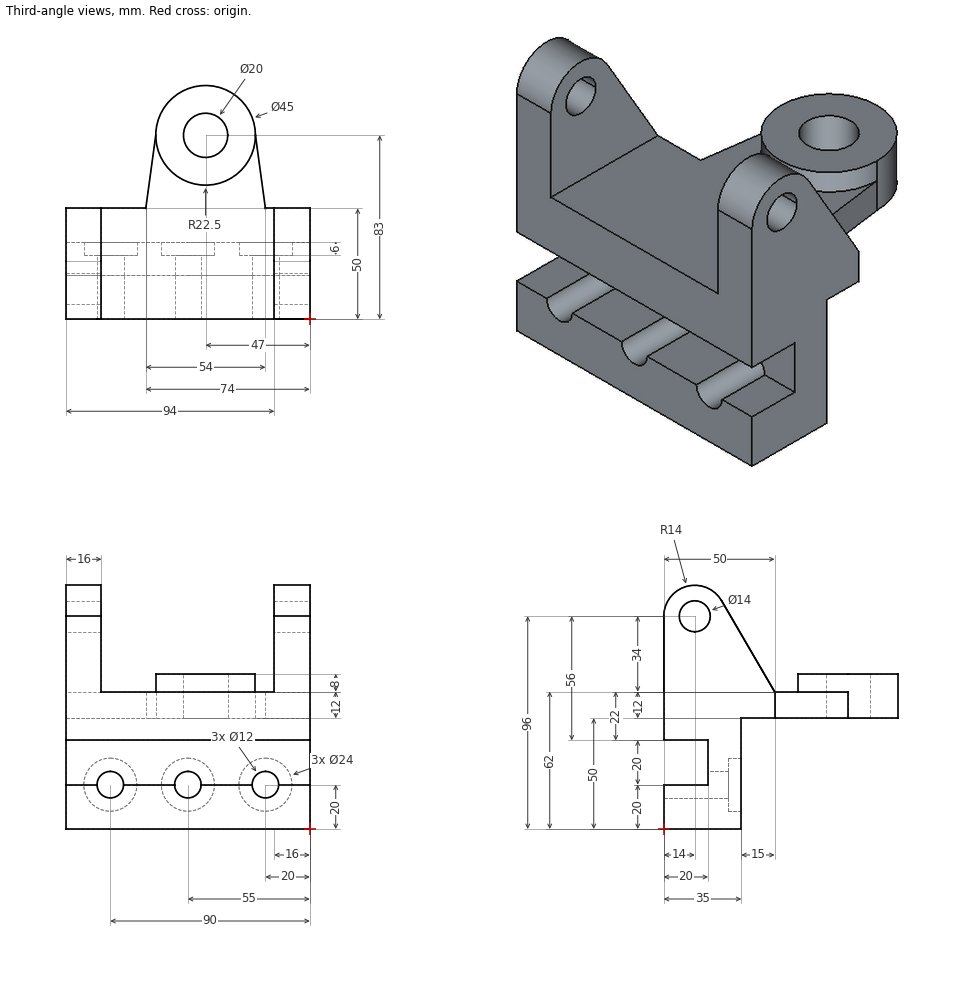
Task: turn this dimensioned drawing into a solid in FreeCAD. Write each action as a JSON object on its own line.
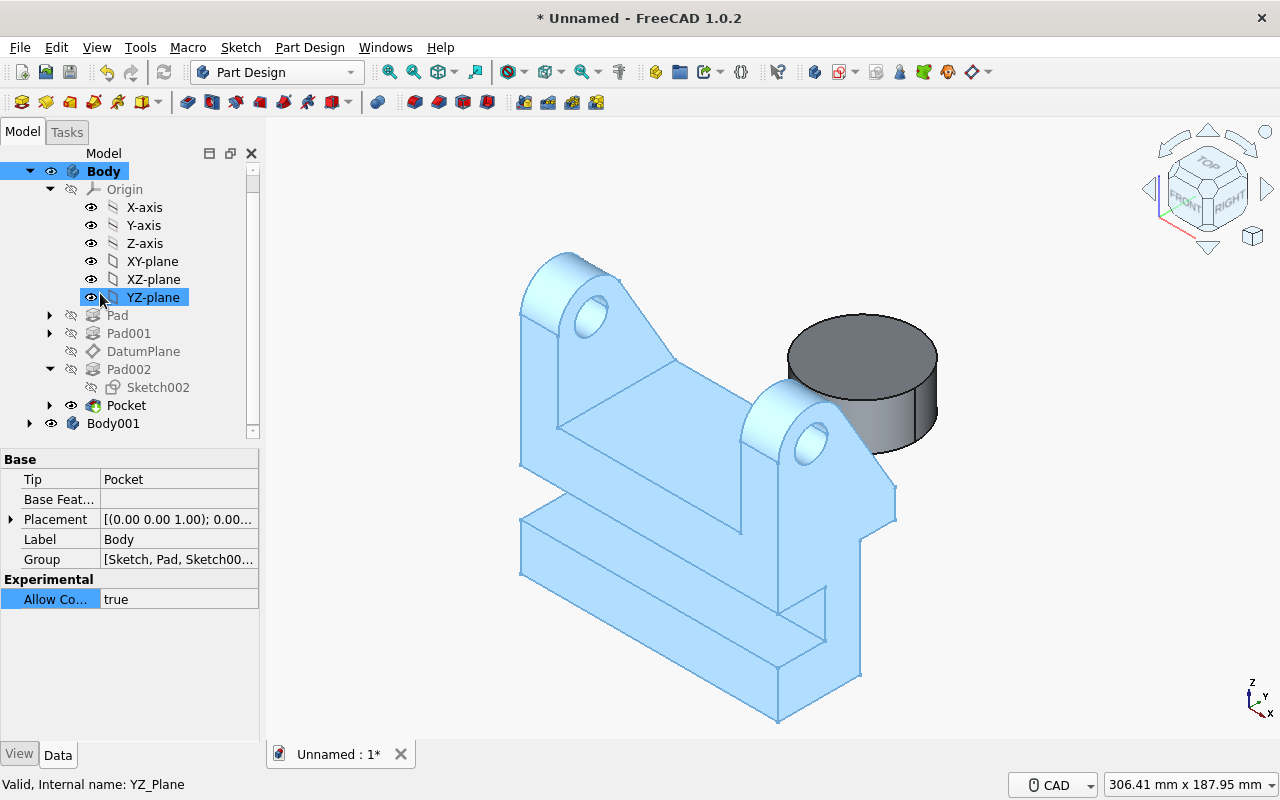
{"action": "left_click", "coordinate": [96, 423]}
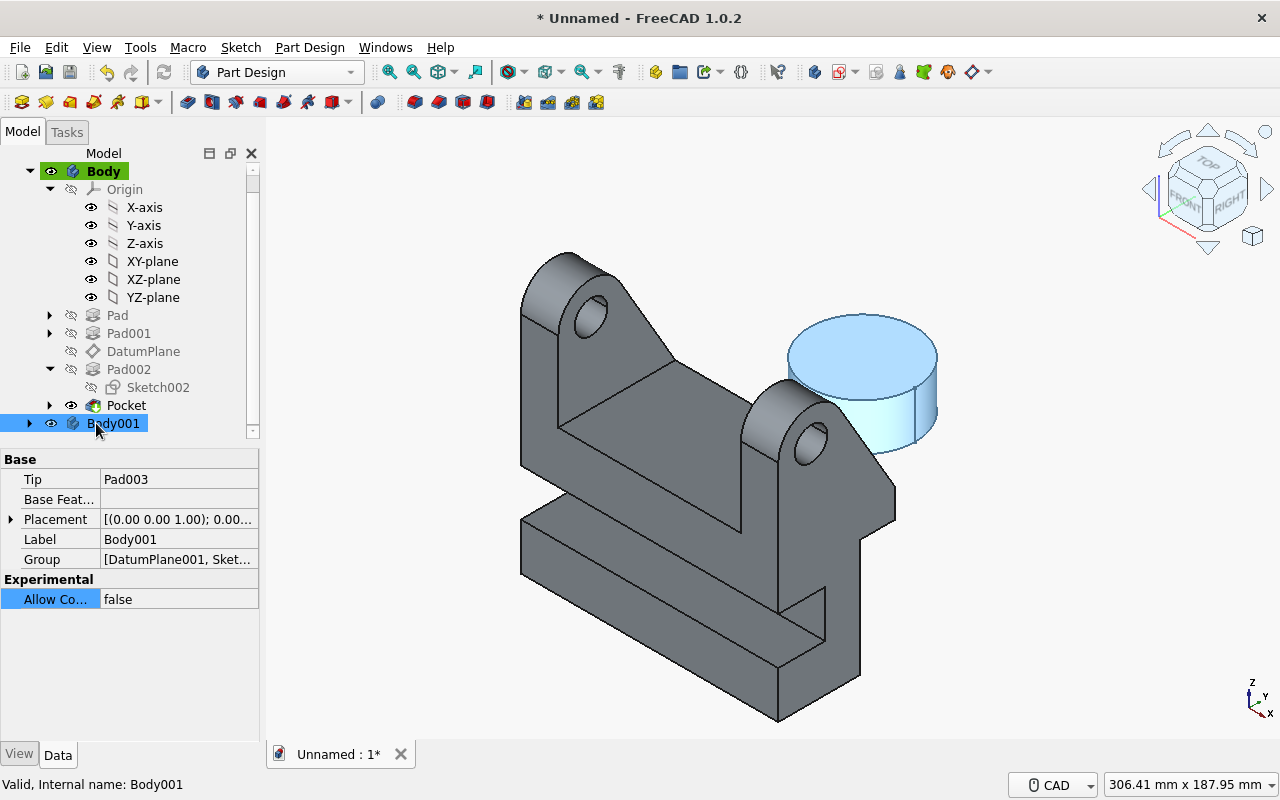
{"action": "left_click", "coordinate": [378, 102]}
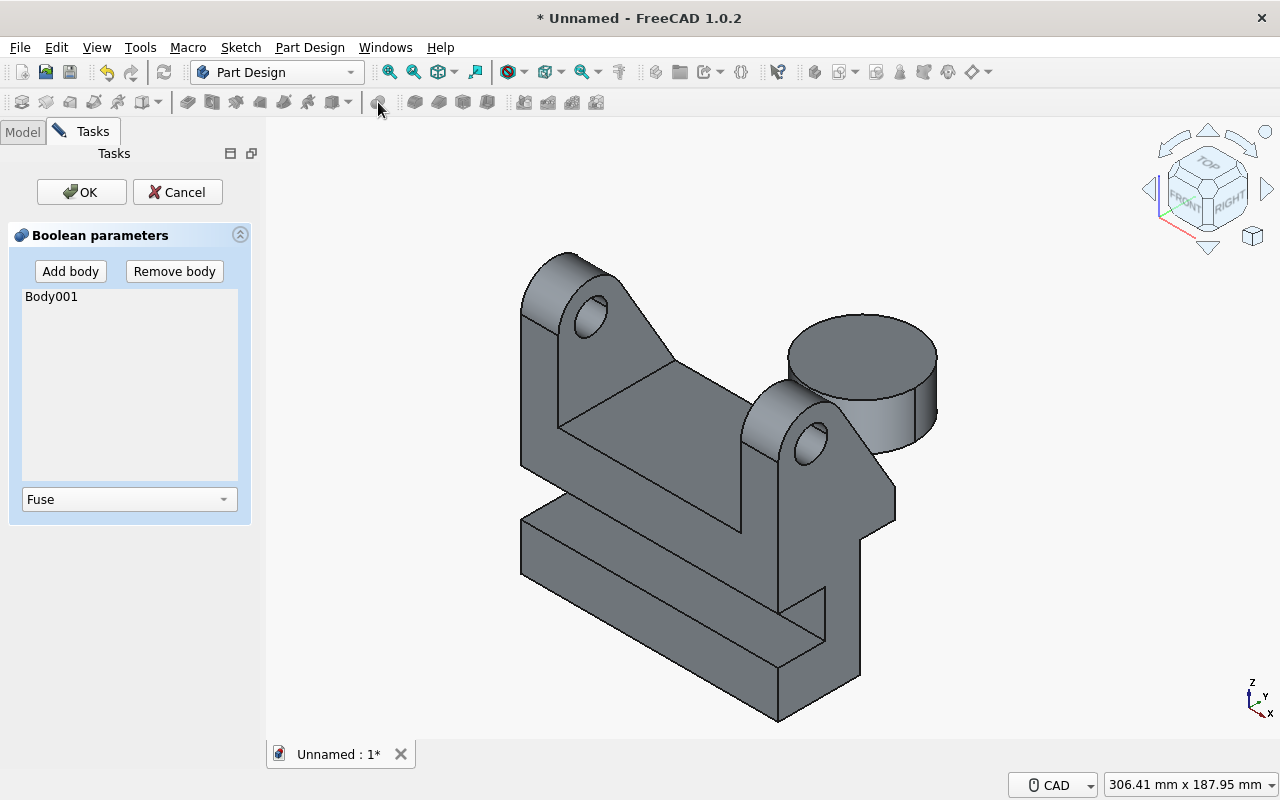
{"action": "left_click", "coordinate": [82, 192]}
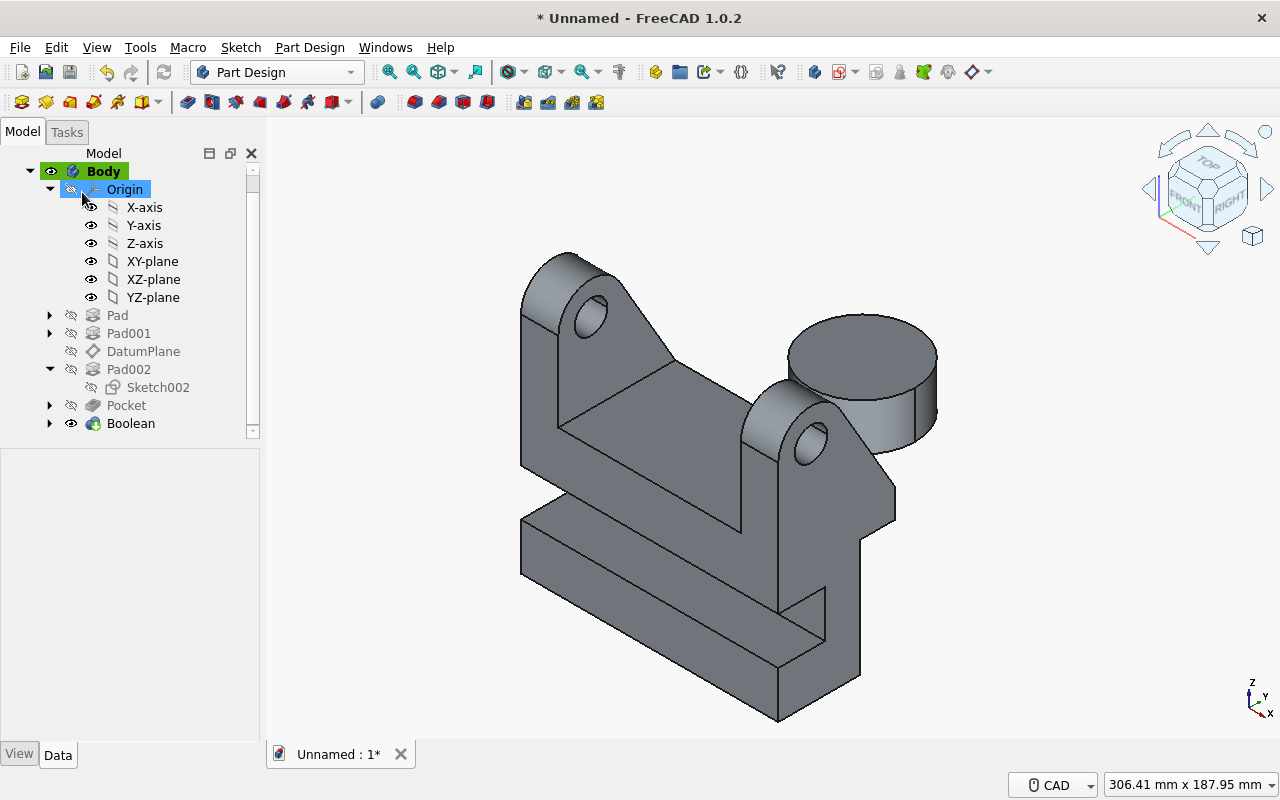
{"action": "left_click", "coordinate": [708, 446]}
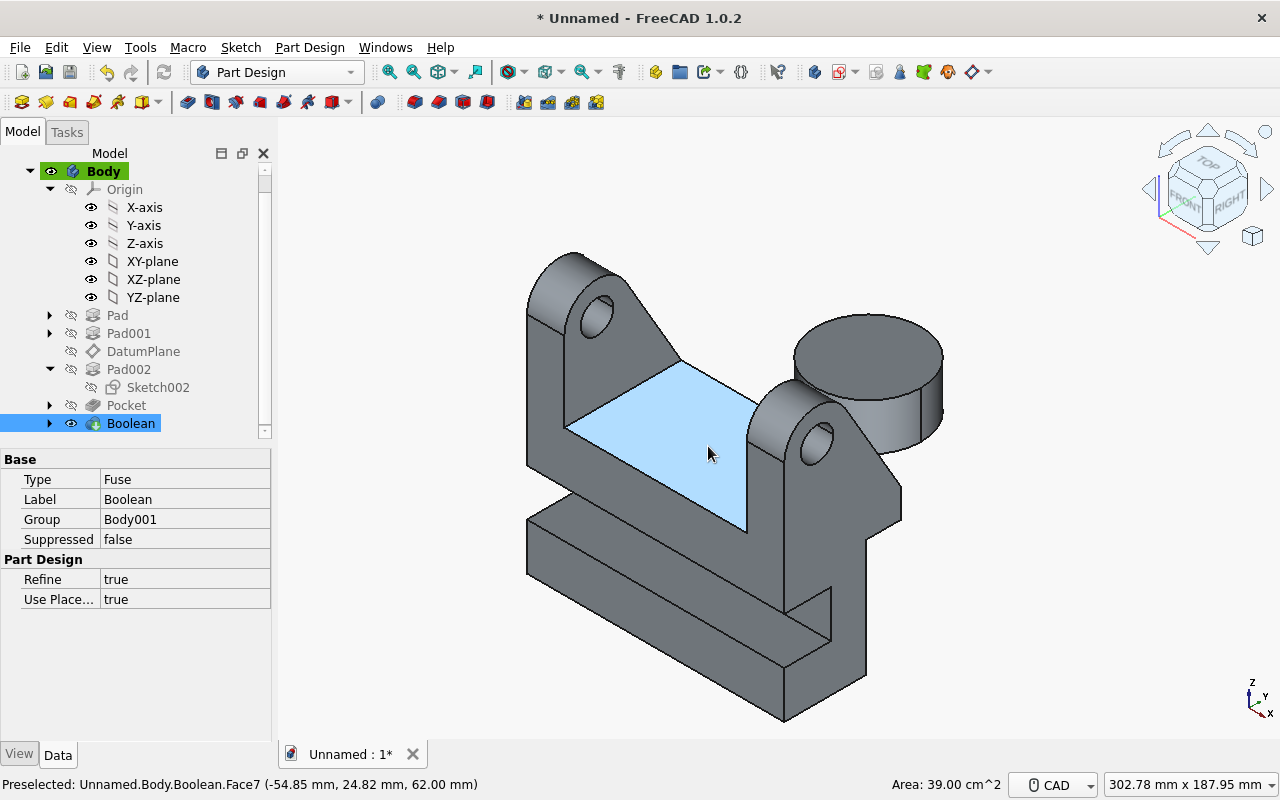
{"action": "left_click", "coordinate": [840, 72]}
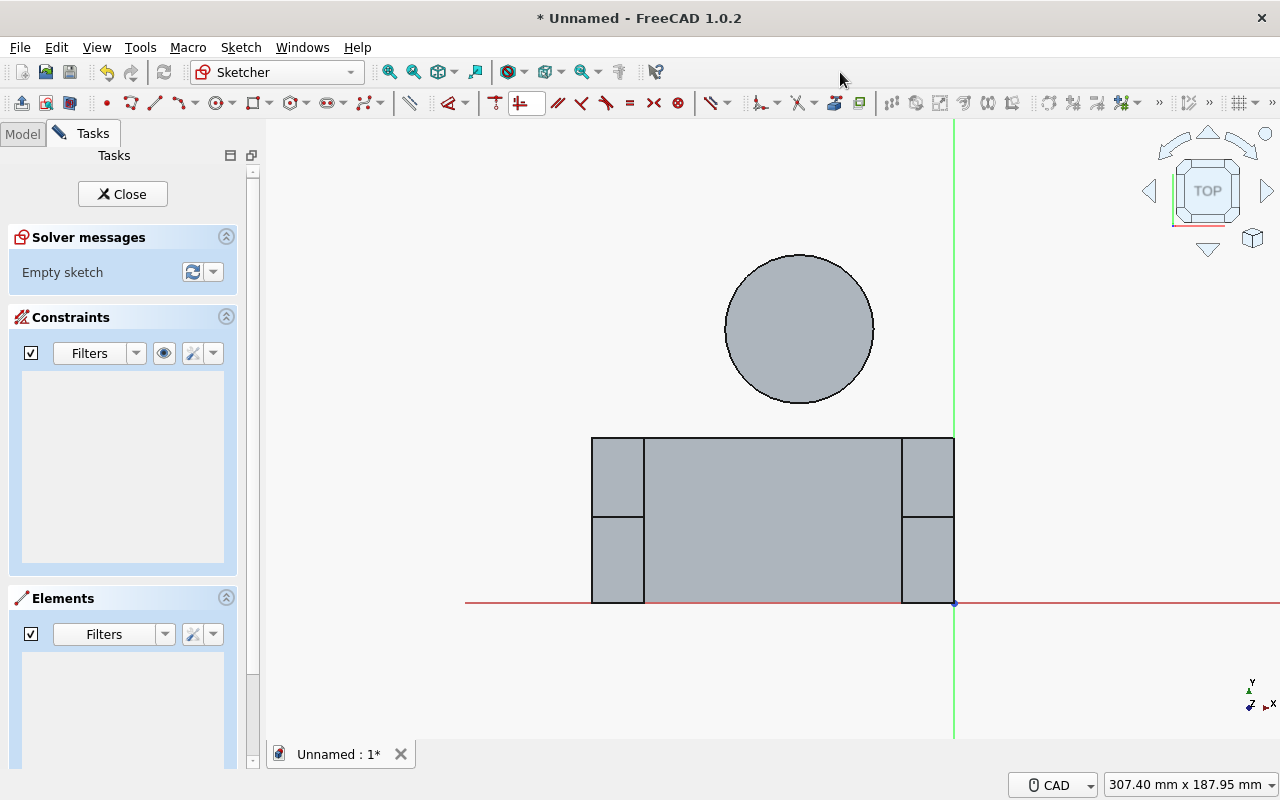
{"action": "left_click", "coordinate": [70, 104]}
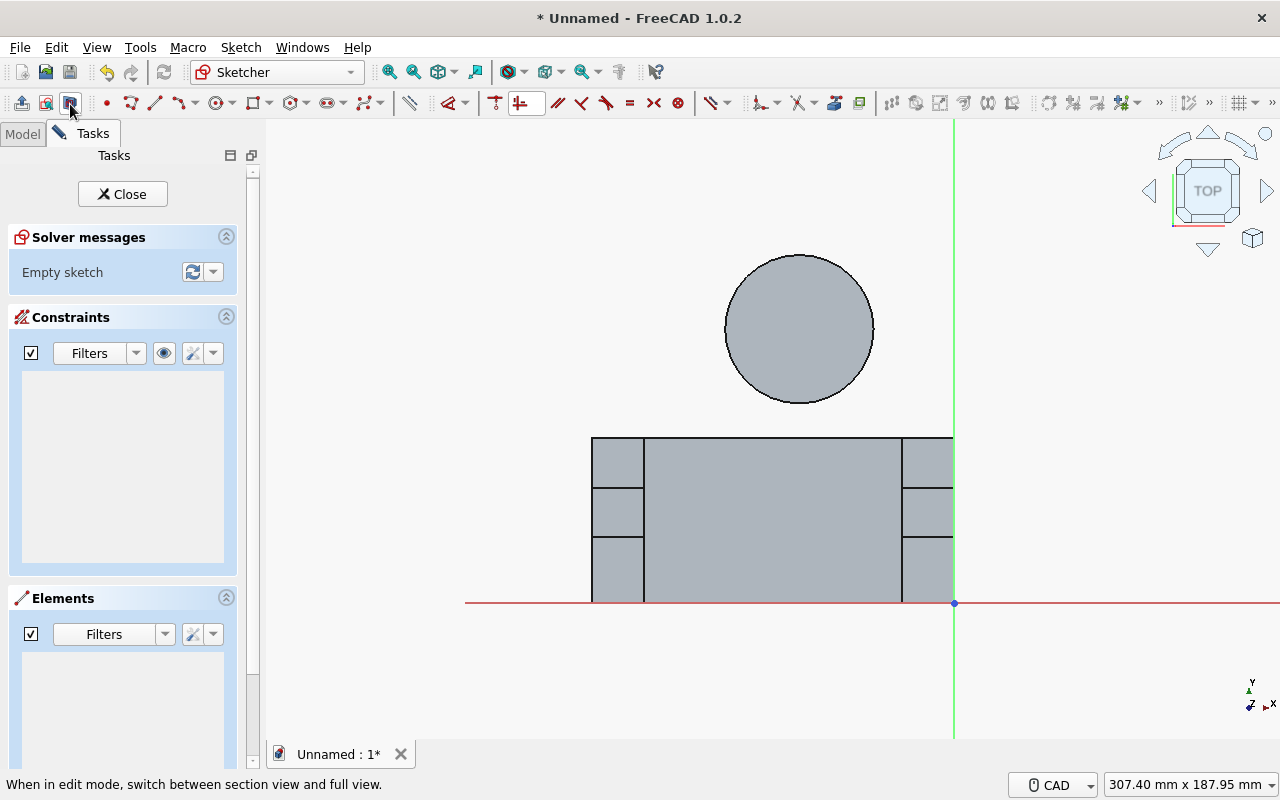
{"action": "scroll", "coordinate": [1092, 542], "scroll_direction": "up", "scroll_amount": 2}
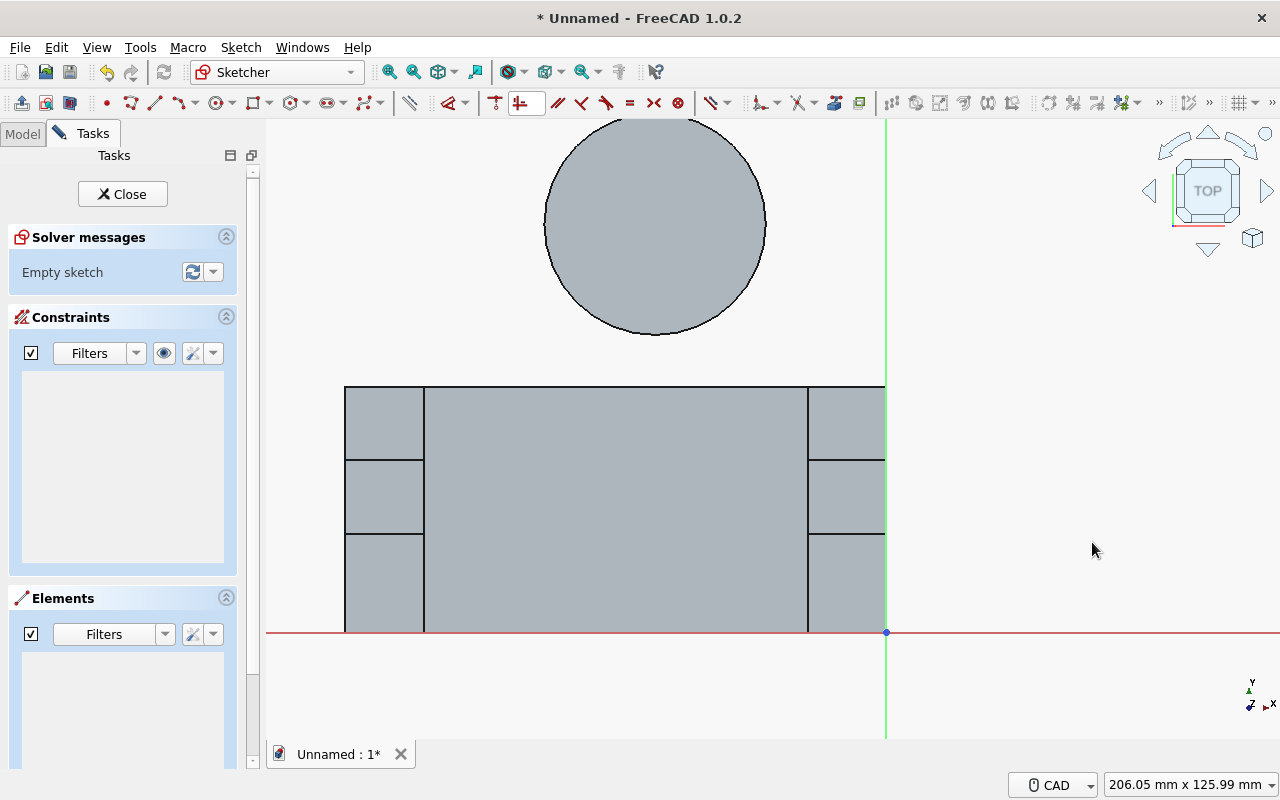
{"action": "left_click", "coordinate": [132, 104]}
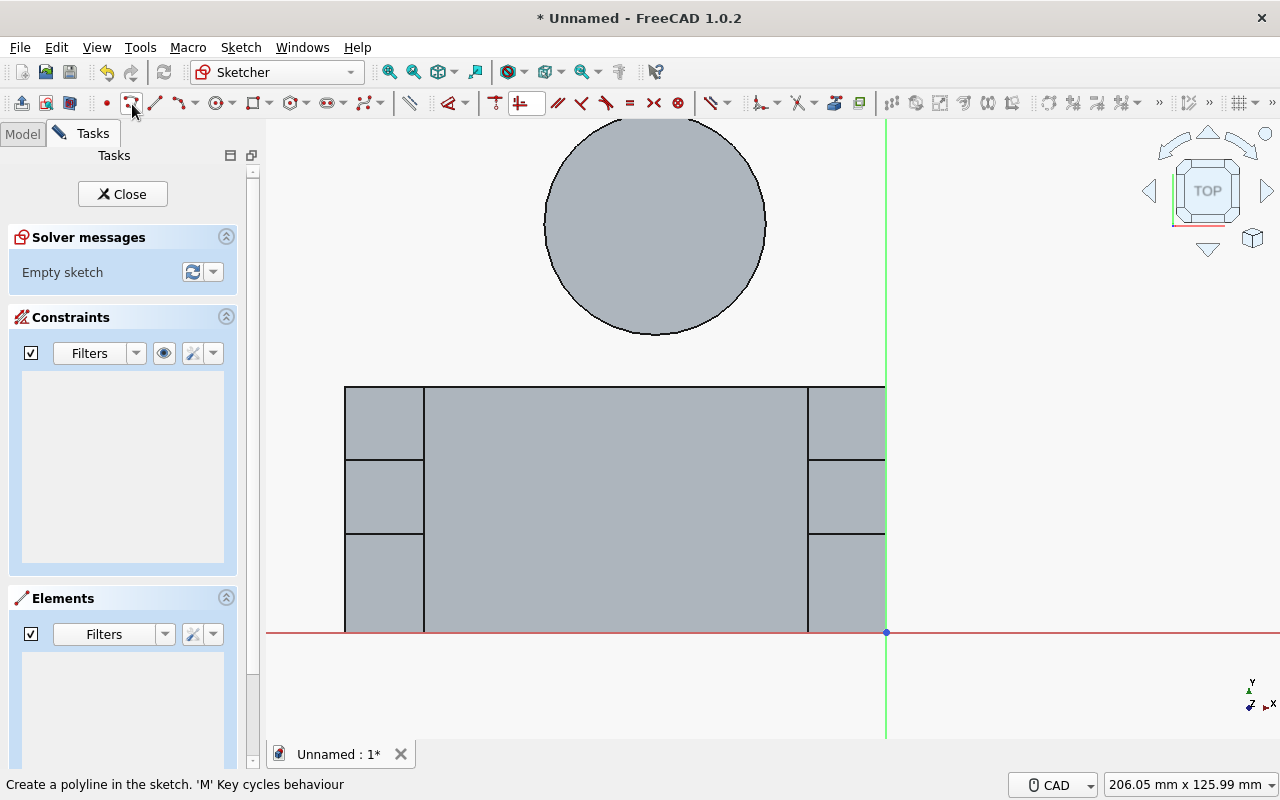
{"action": "left_click", "coordinate": [544, 224]}
{"action": "left_click", "coordinate": [522, 387]}
{"action": "left_click", "coordinate": [788, 387]}
{"action": "left_click", "coordinate": [766, 224]}
{"action": "right_click", "coordinate": [766, 224]}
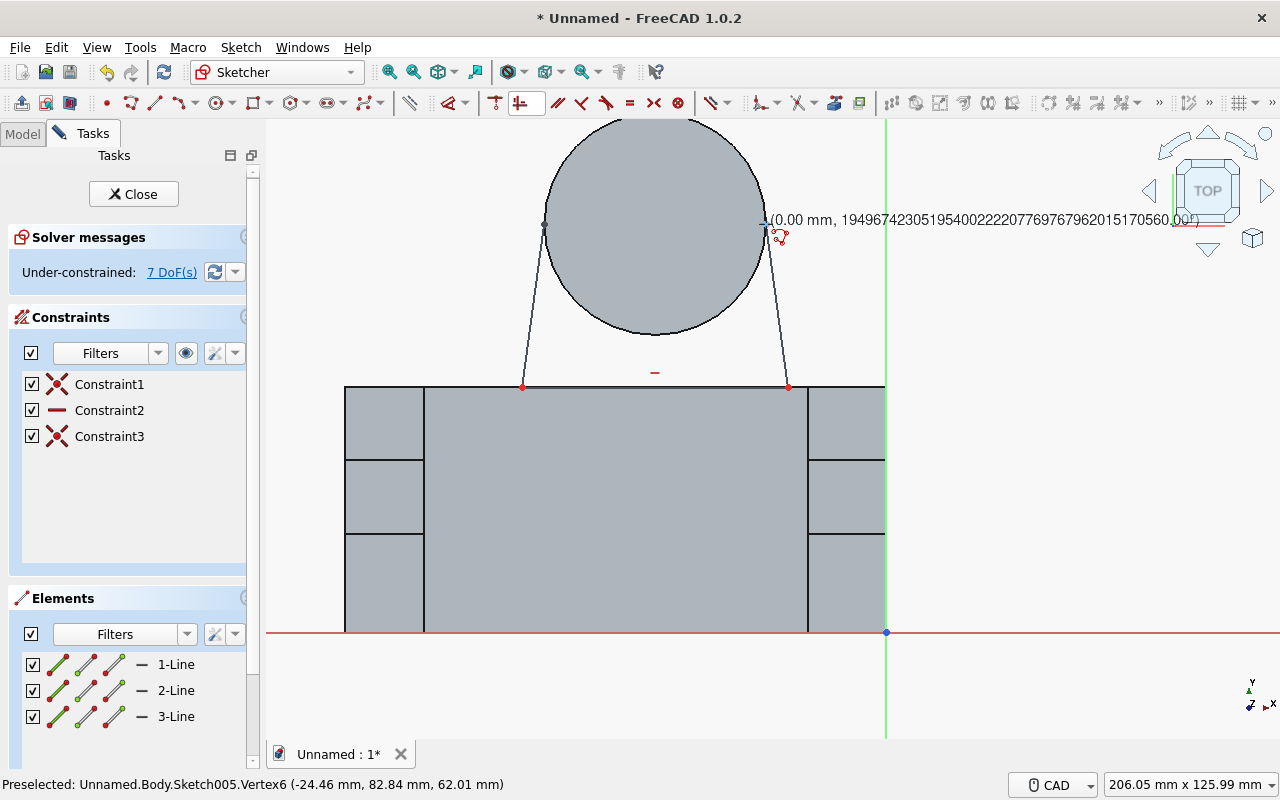
{"action": "left_click", "coordinate": [180, 104]}